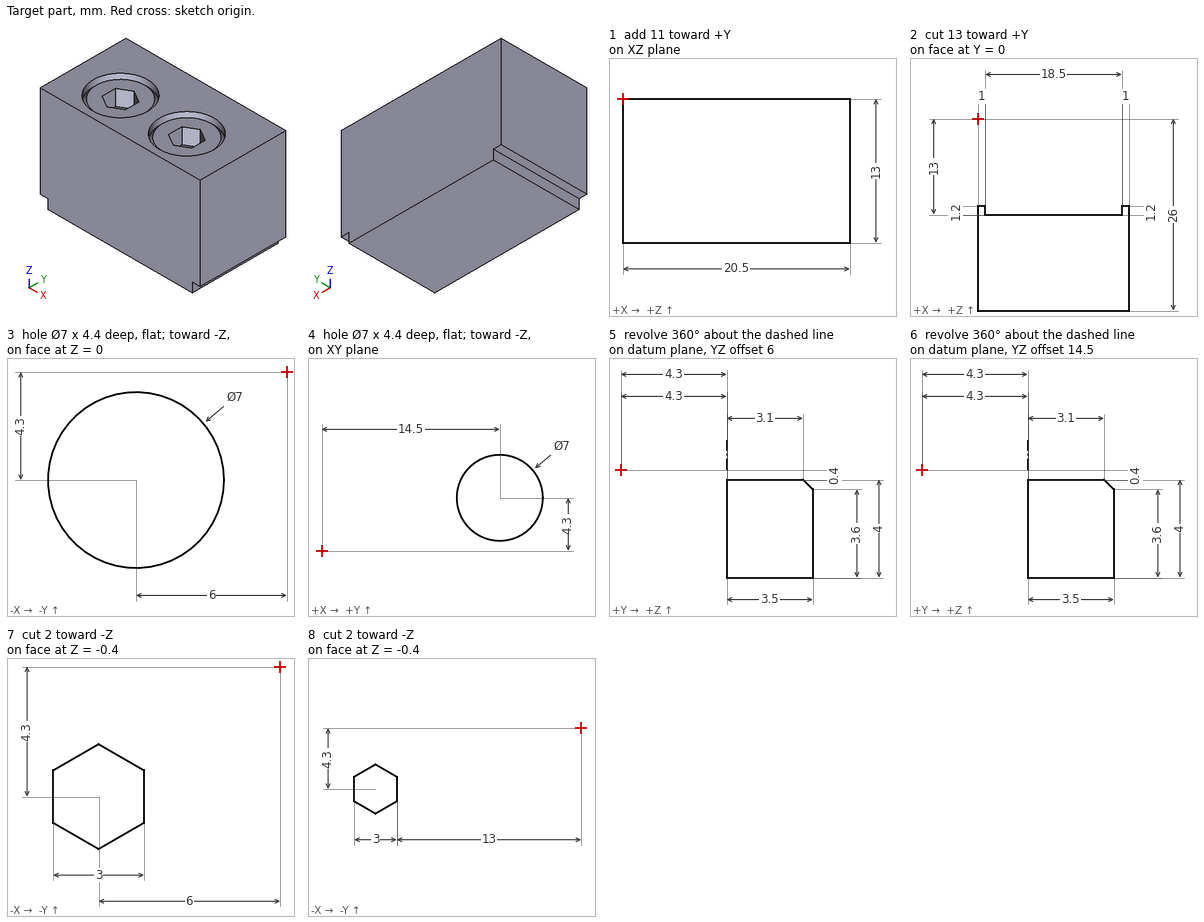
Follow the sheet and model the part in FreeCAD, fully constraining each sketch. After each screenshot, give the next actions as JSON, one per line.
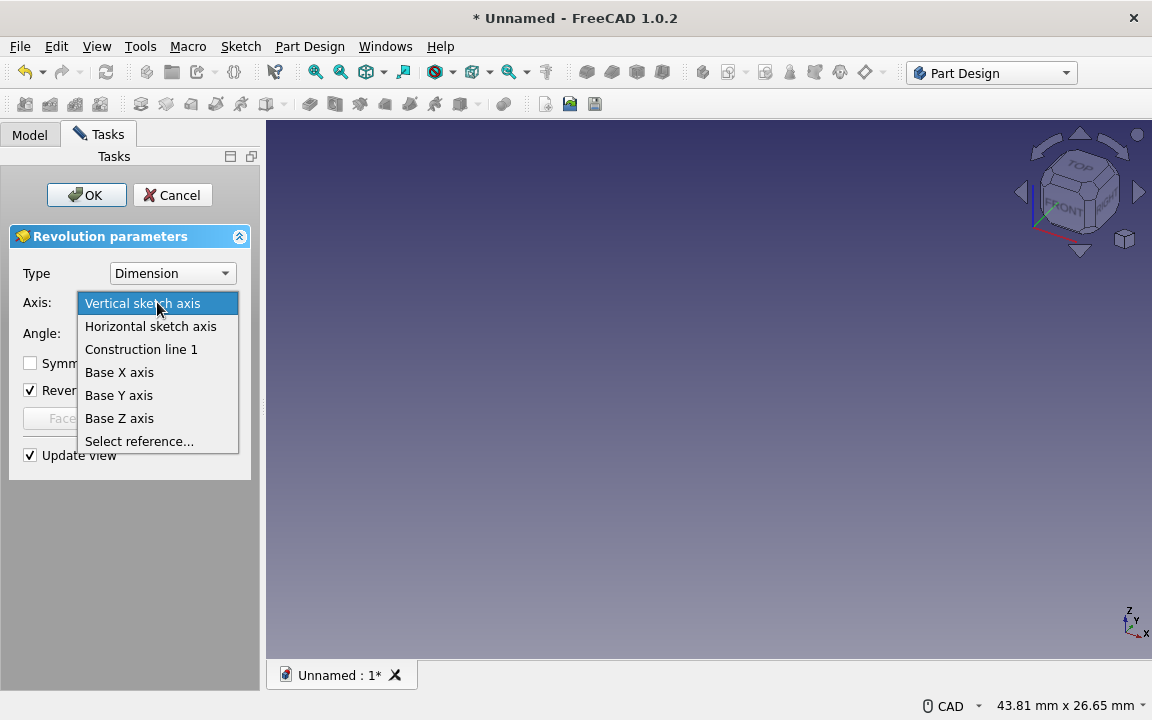
{"action": "left_click", "coordinate": [156, 350]}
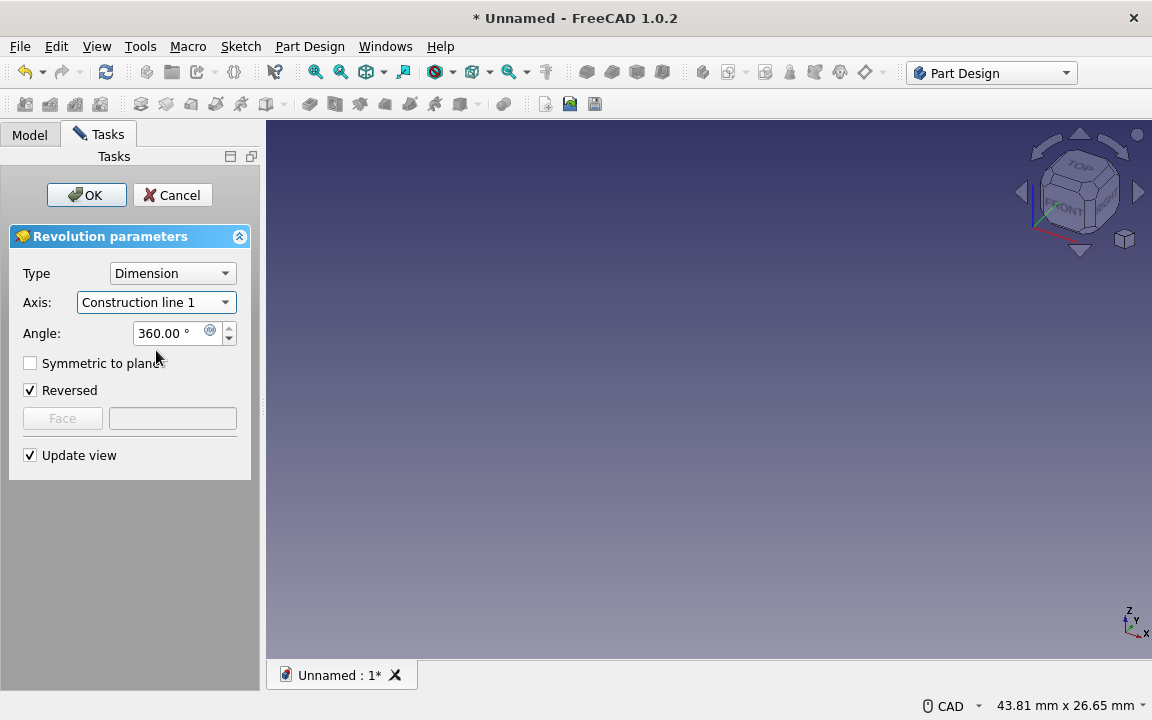
{"action": "left_click", "coordinate": [87, 195]}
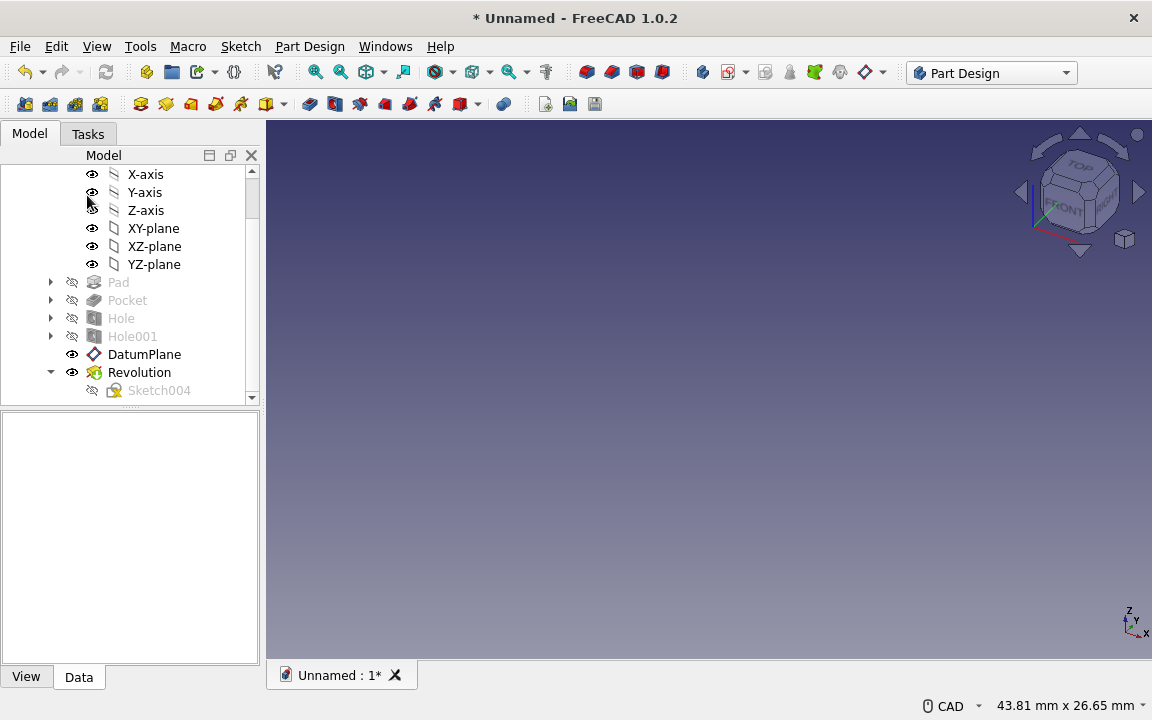
{"action": "left_click", "coordinate": [117, 354]}
{"action": "key", "text": "space"}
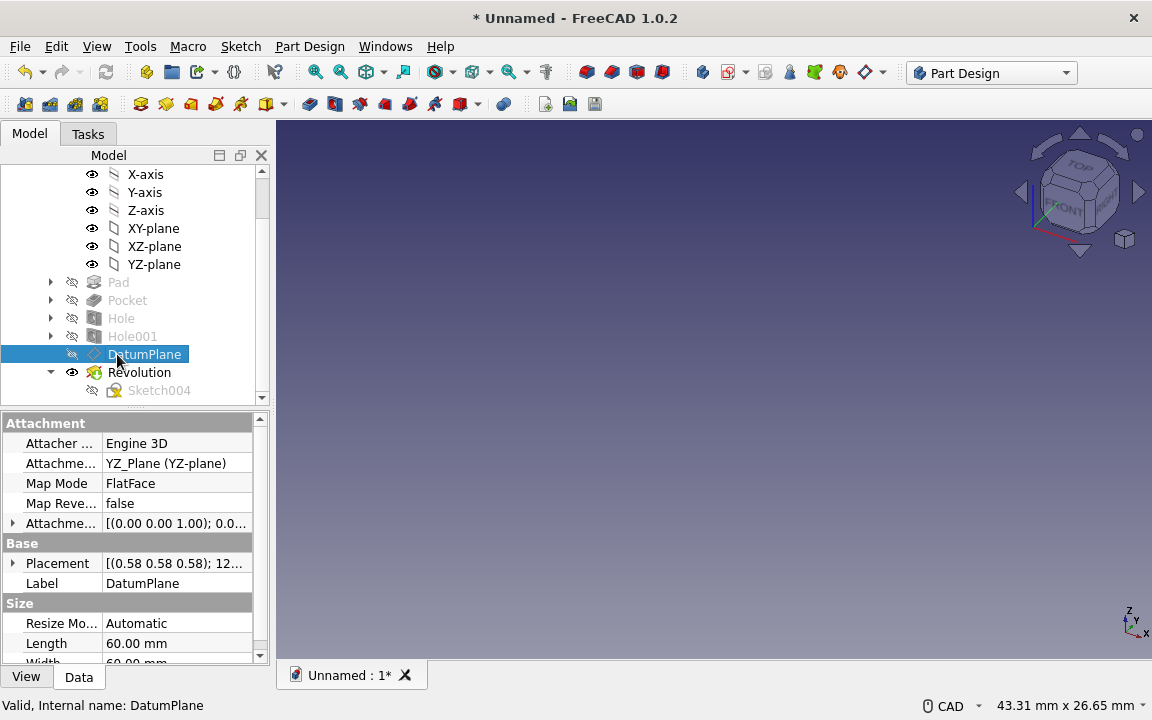
{"action": "left_click", "coordinate": [316, 72]}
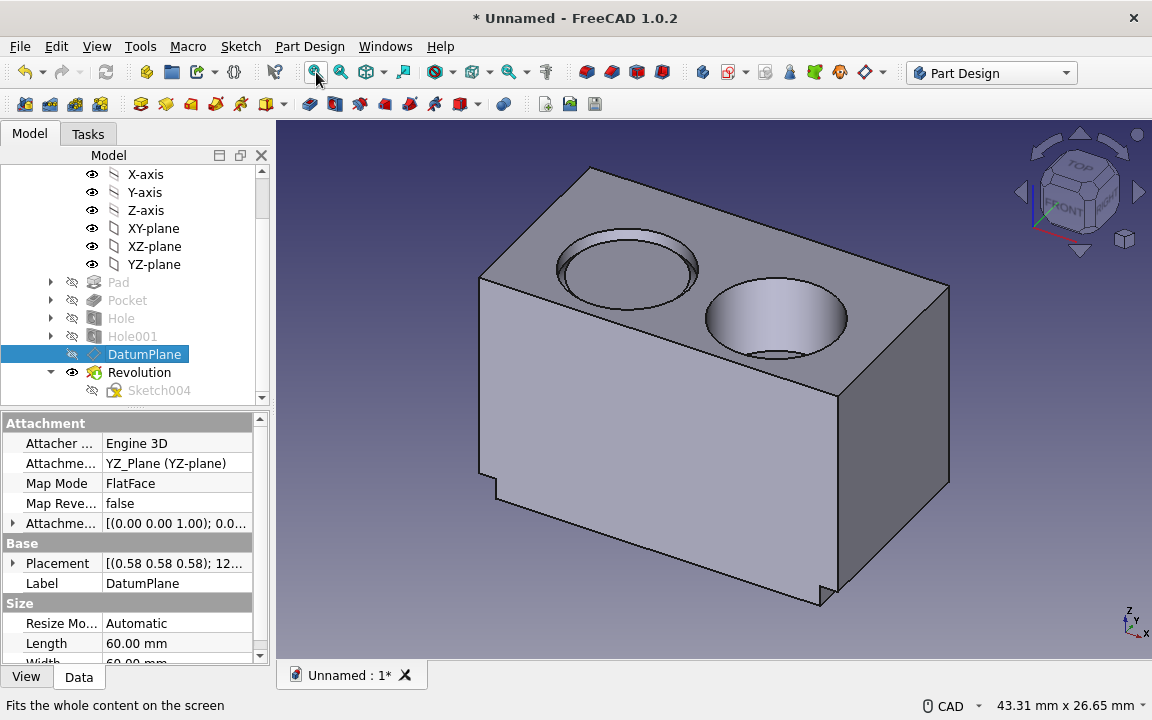
{"action": "scroll", "coordinate": [161, 278], "scroll_direction": "down", "scroll_amount": 3}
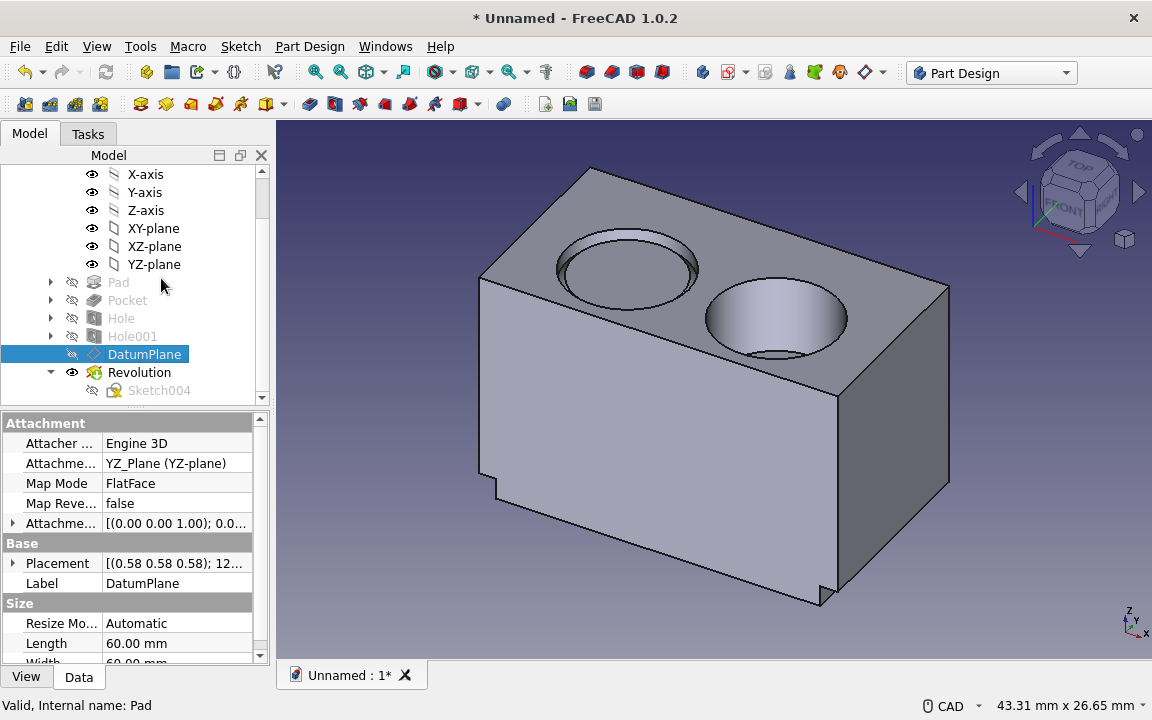
{"action": "scroll", "coordinate": [161, 278], "scroll_direction": "up", "scroll_amount": 15}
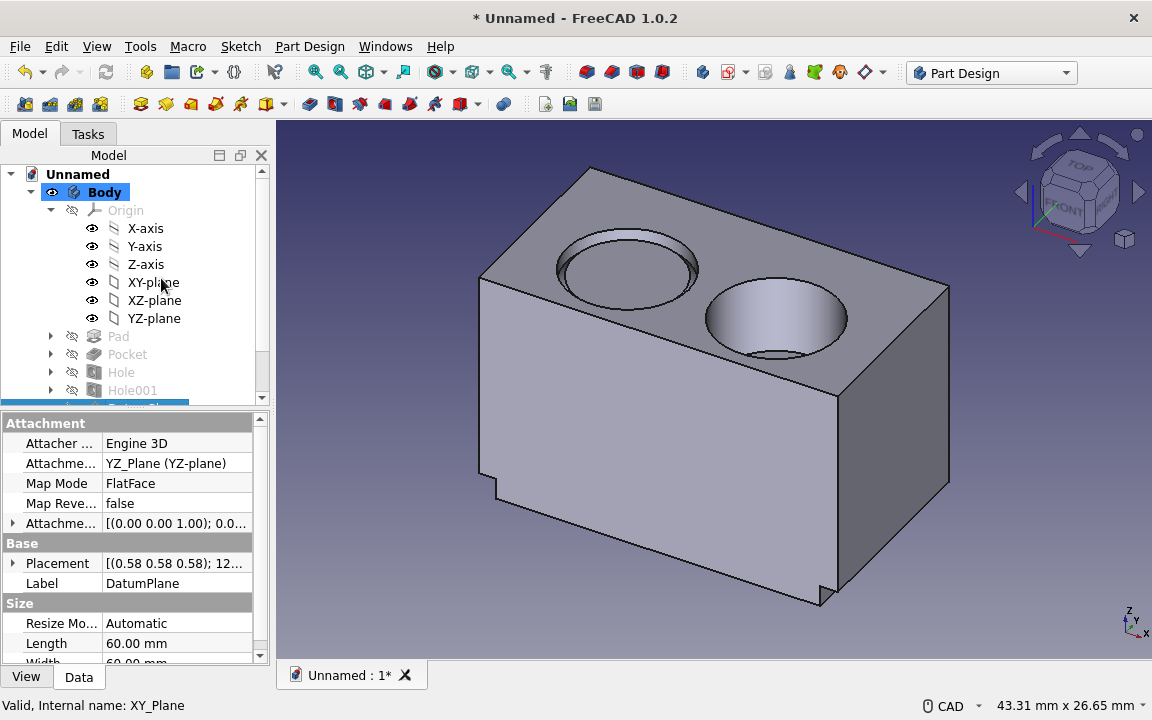
{"action": "left_click", "coordinate": [137, 318]}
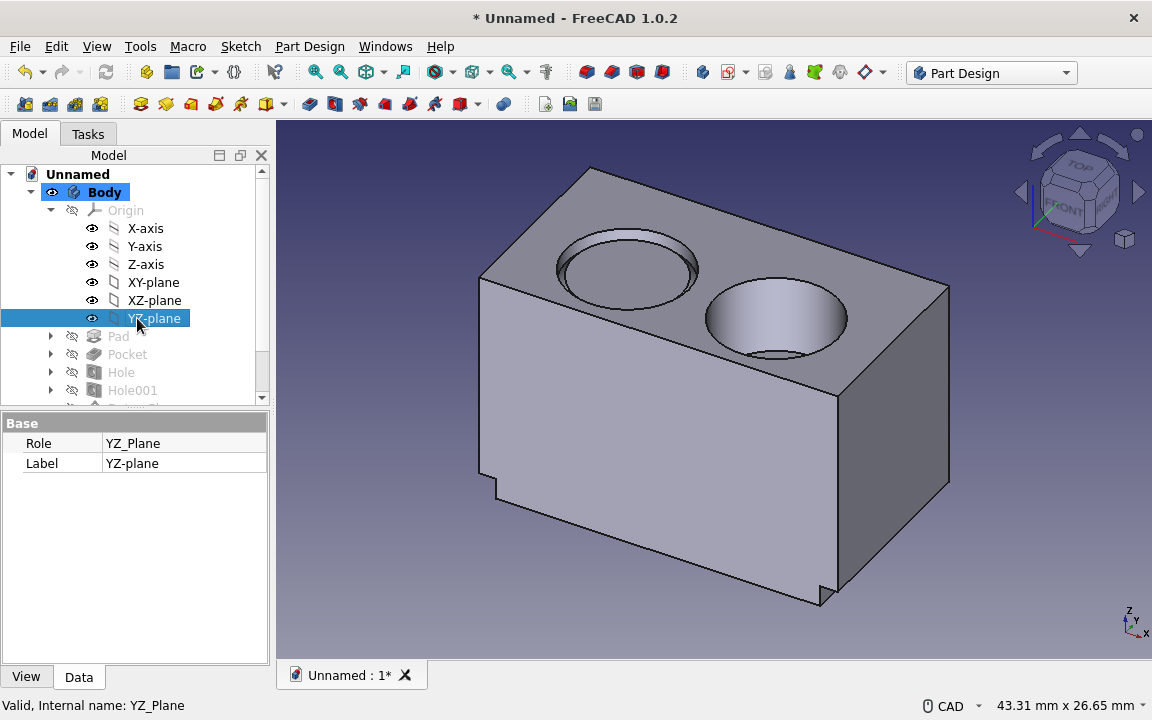
{"action": "left_click", "coordinate": [864, 72]}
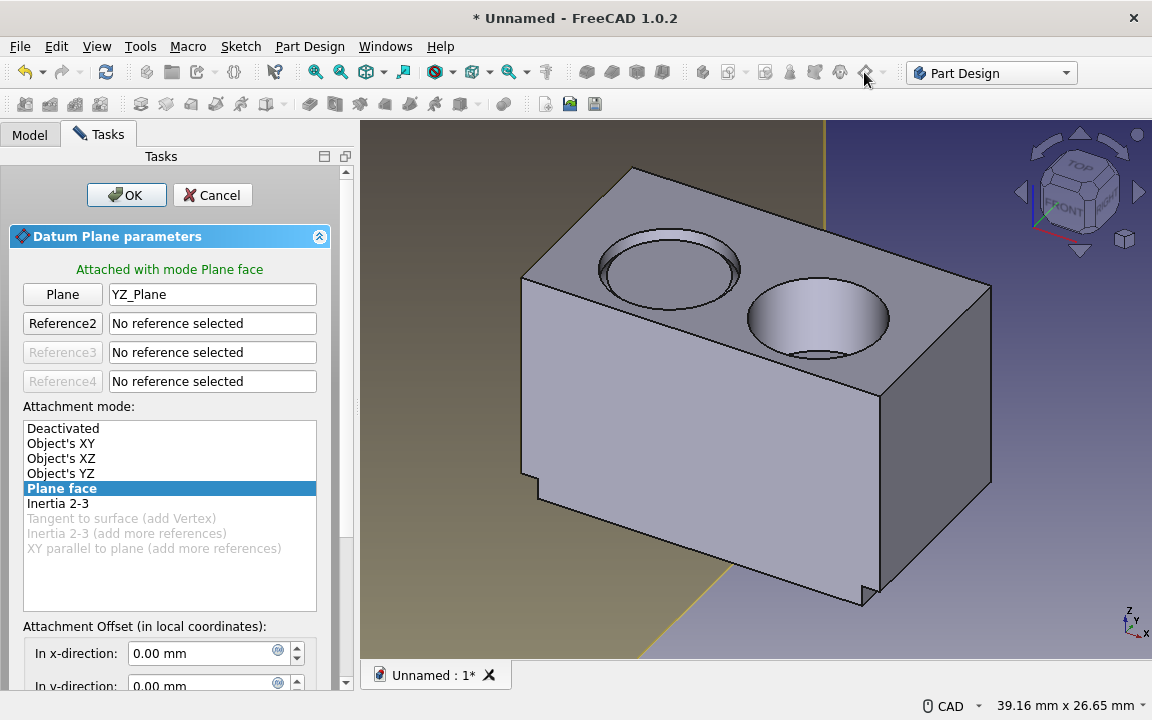
{"action": "scroll", "coordinate": [346, 428], "scroll_direction": "down", "scroll_amount": 2}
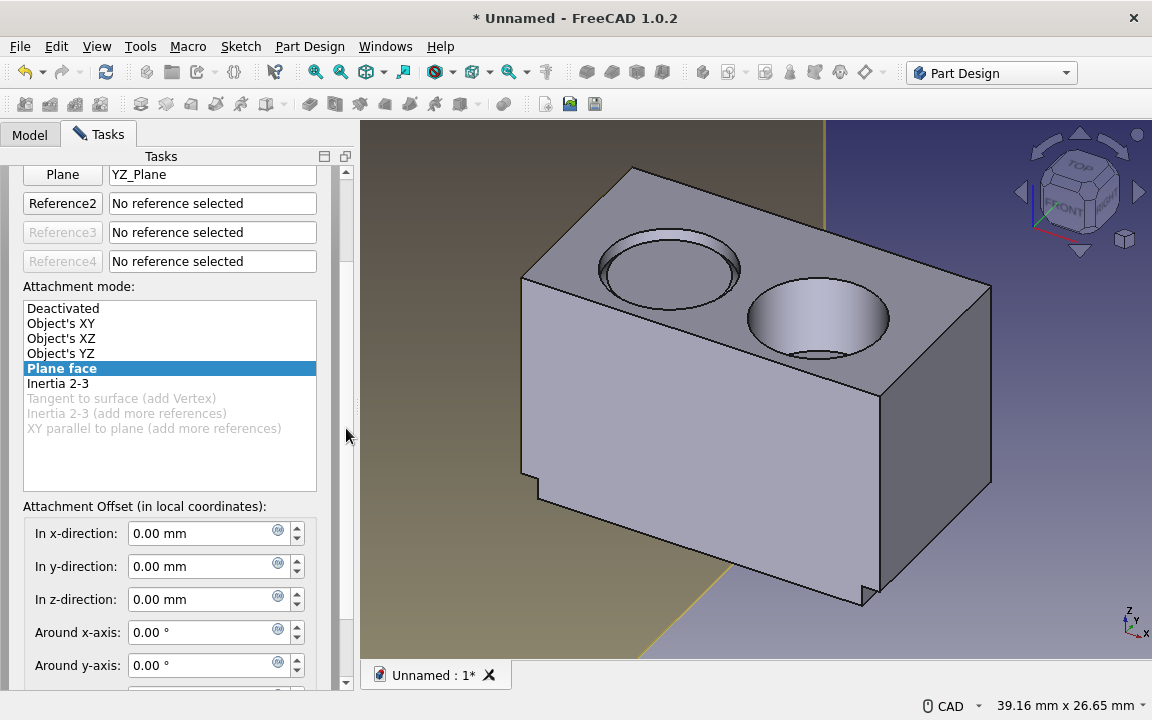
{"action": "triple_click", "coordinate": [210, 600]}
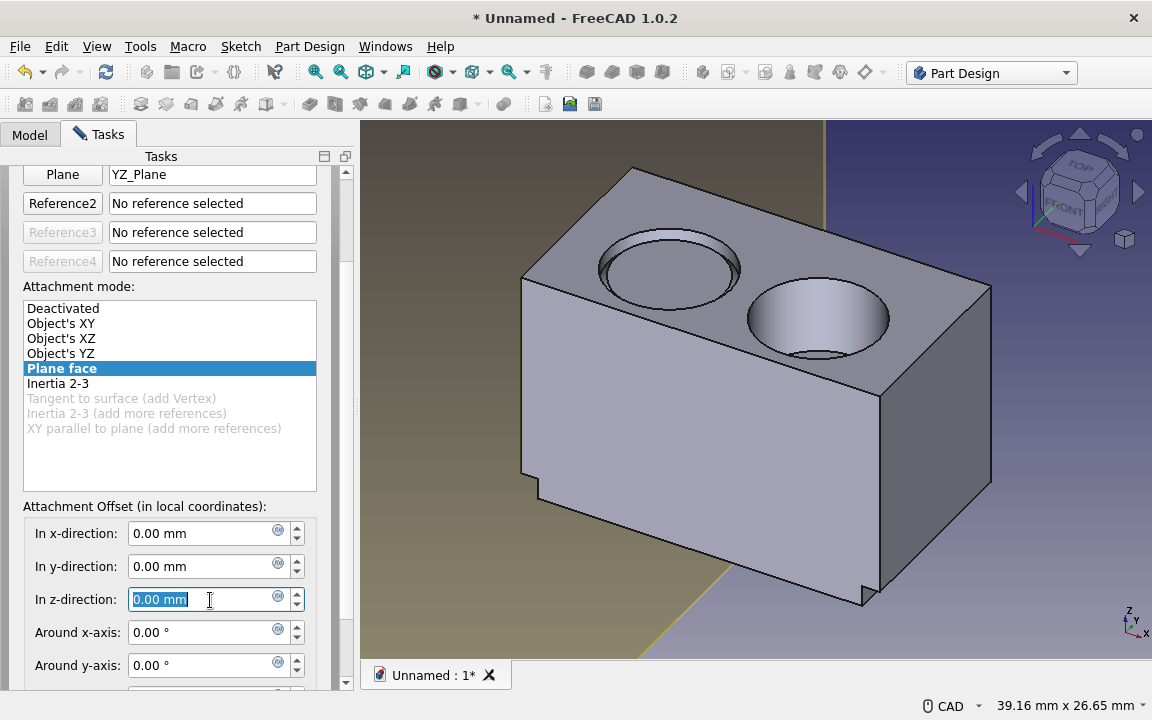
{"action": "type", "text": "14.5"}
{"action": "key", "text": "Tab"}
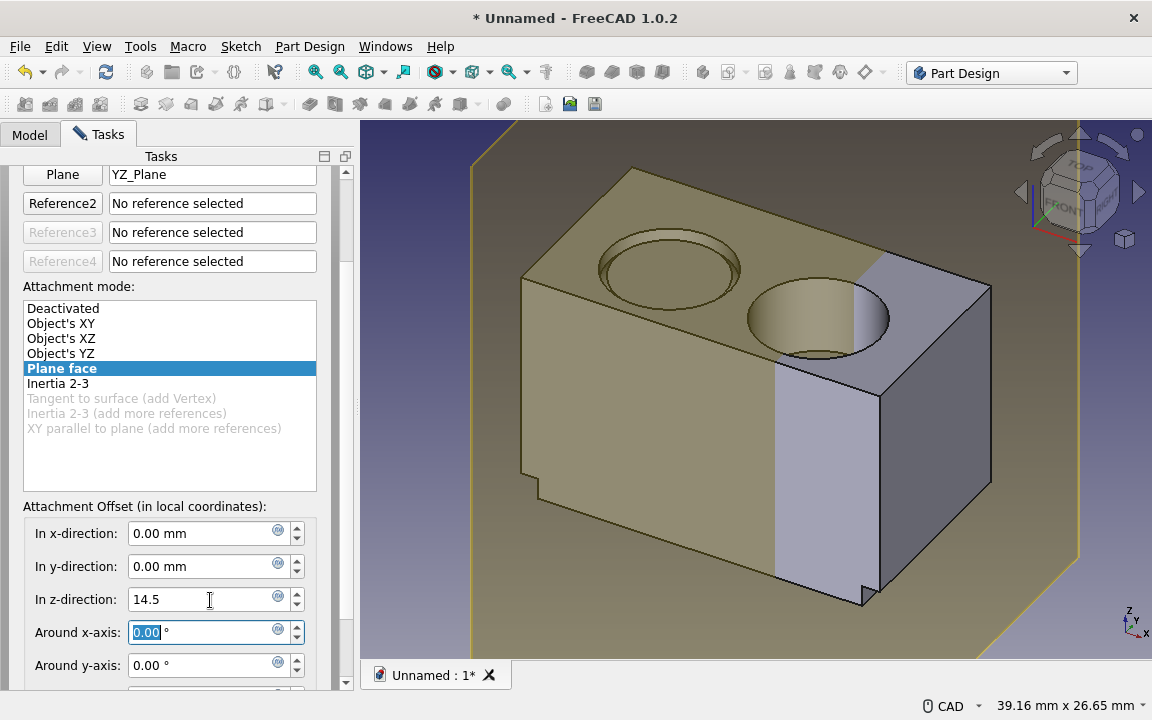
{"action": "scroll", "coordinate": [346, 428], "scroll_direction": "up", "scroll_amount": 3}